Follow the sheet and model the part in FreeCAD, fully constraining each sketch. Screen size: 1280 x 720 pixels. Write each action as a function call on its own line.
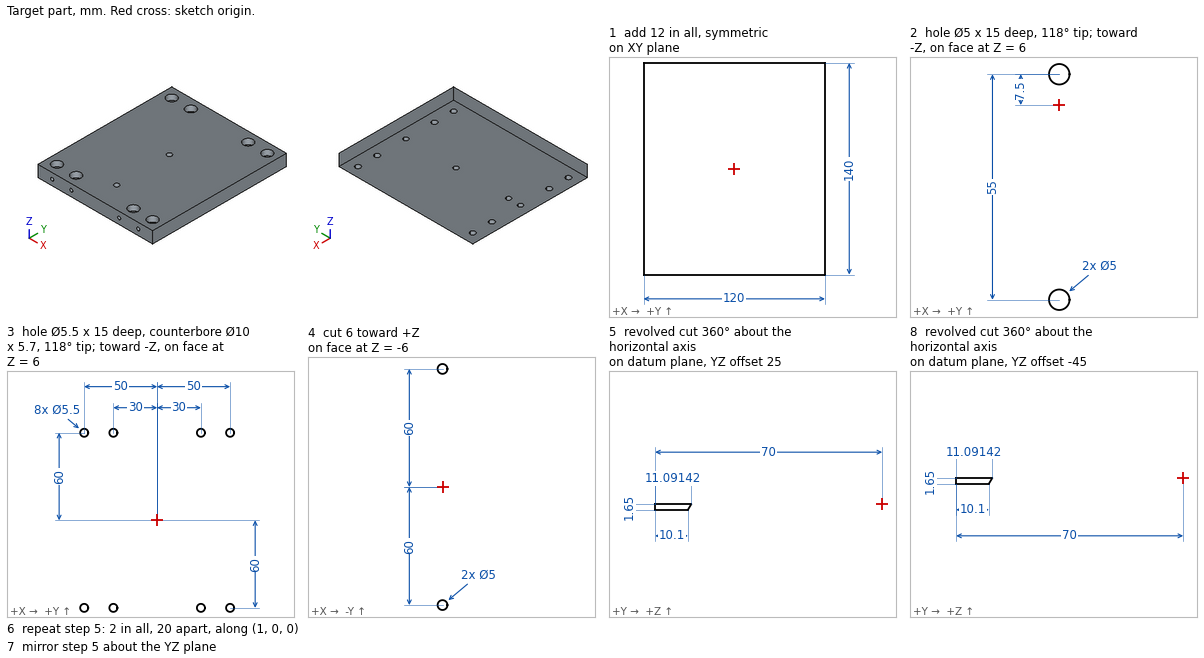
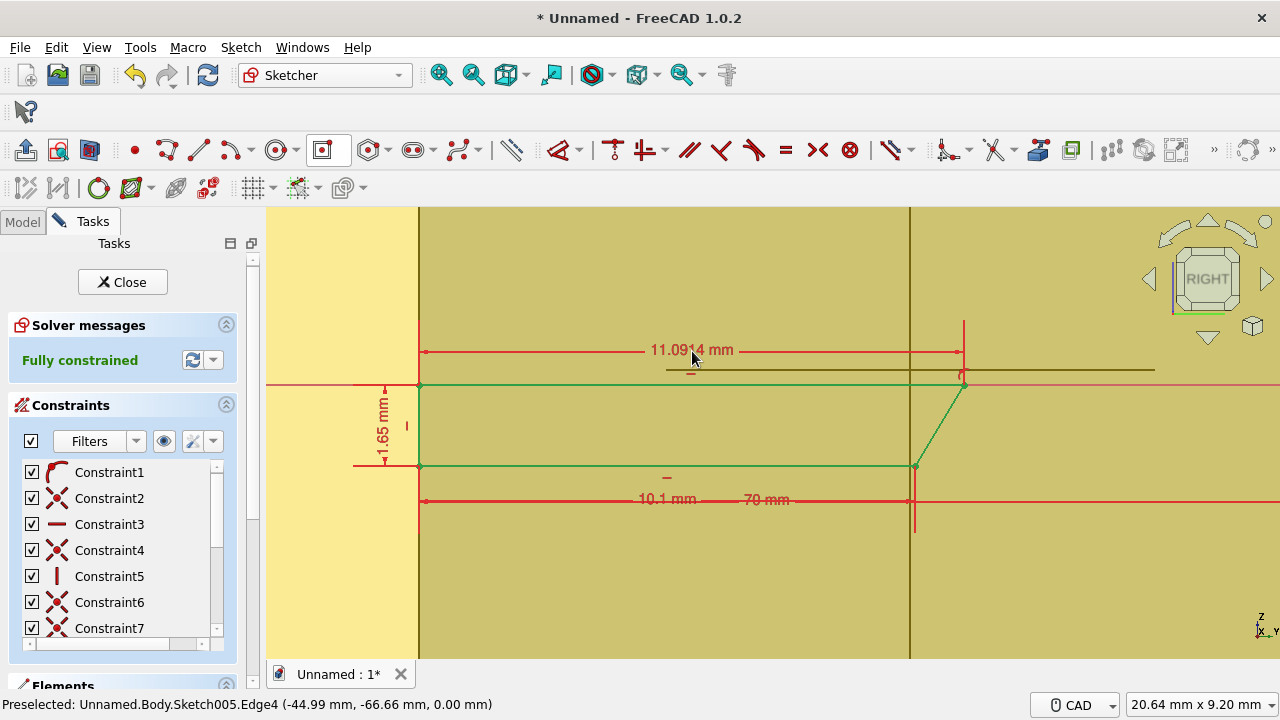
click(123, 282)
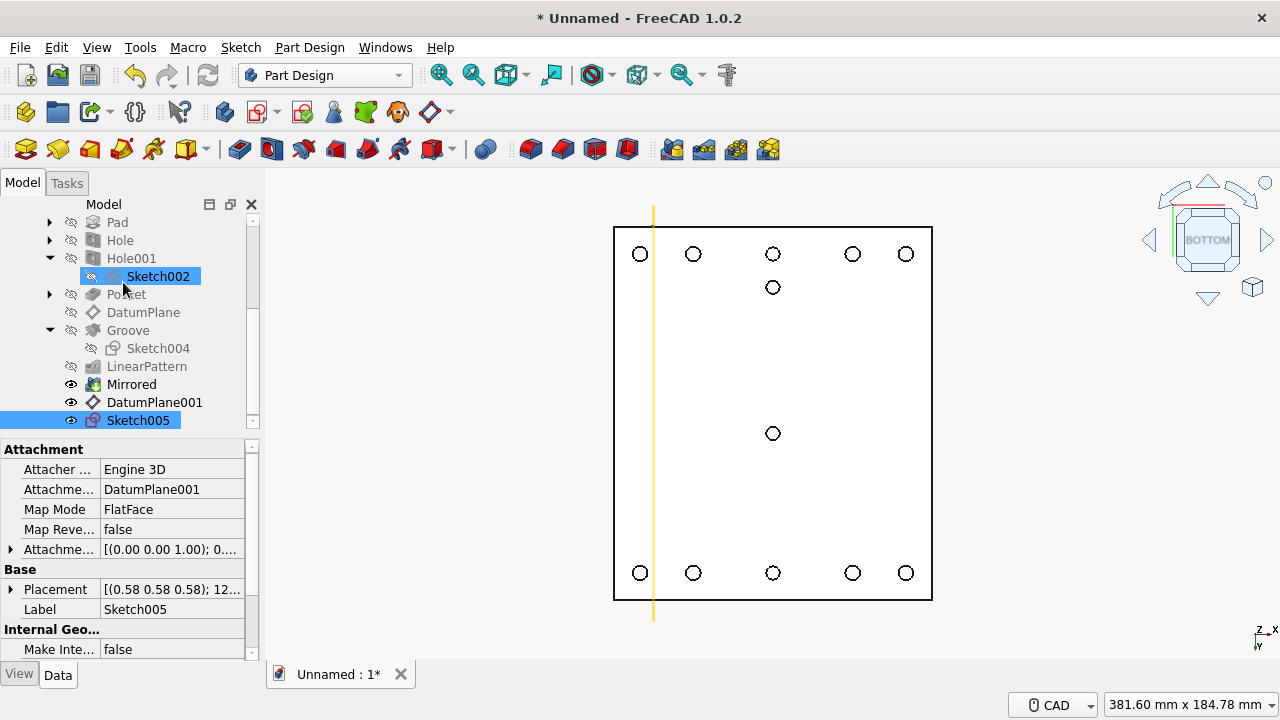
click(304, 150)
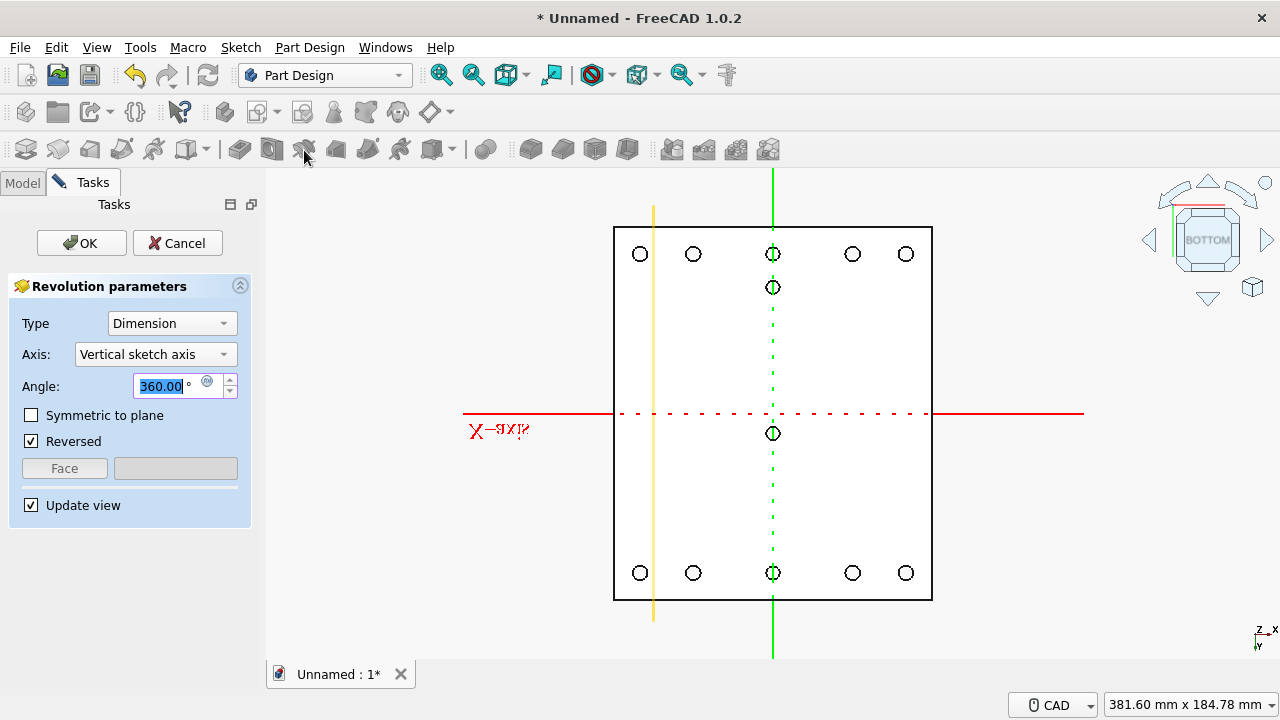
click(156, 354)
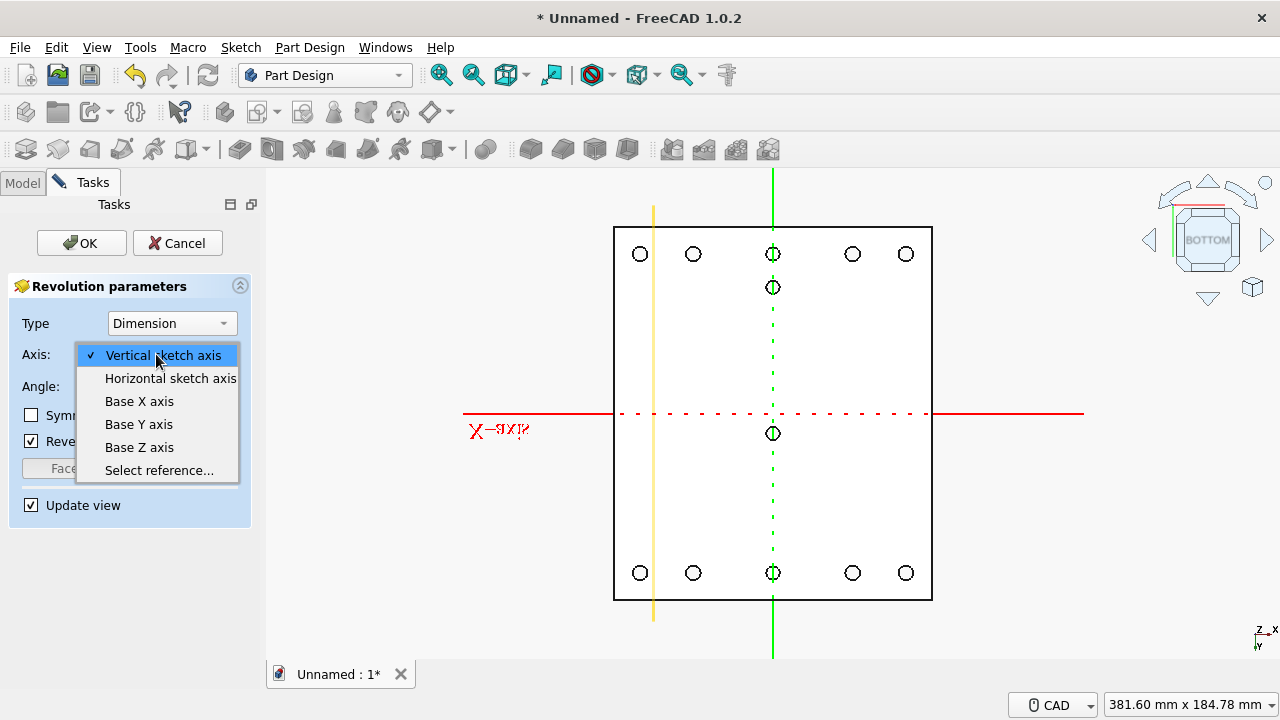
click(156, 378)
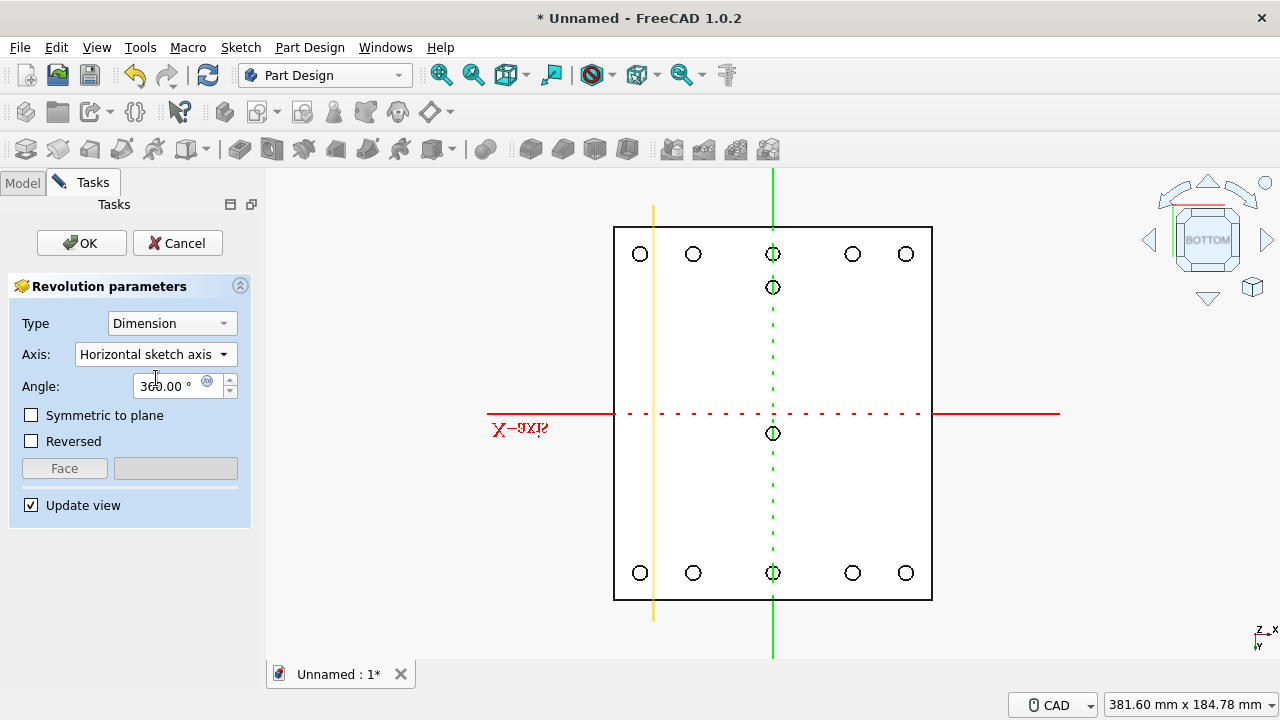
click(82, 243)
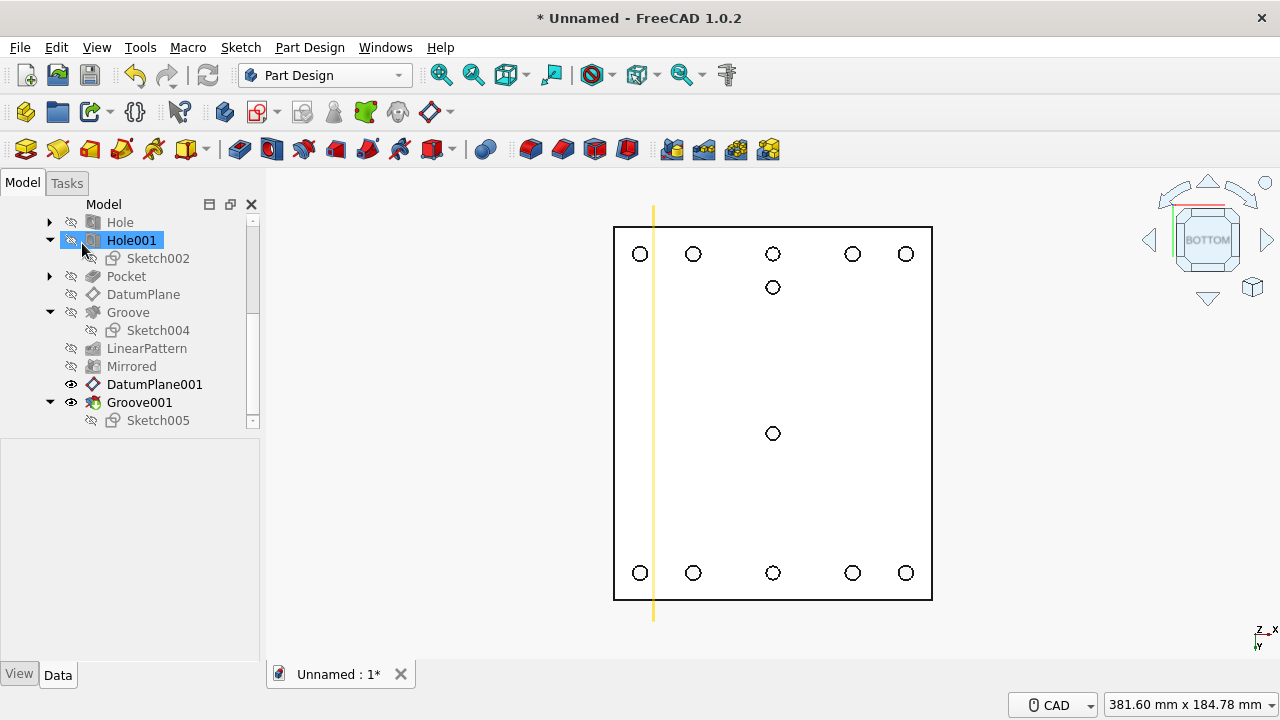
click(116, 384)
key(space)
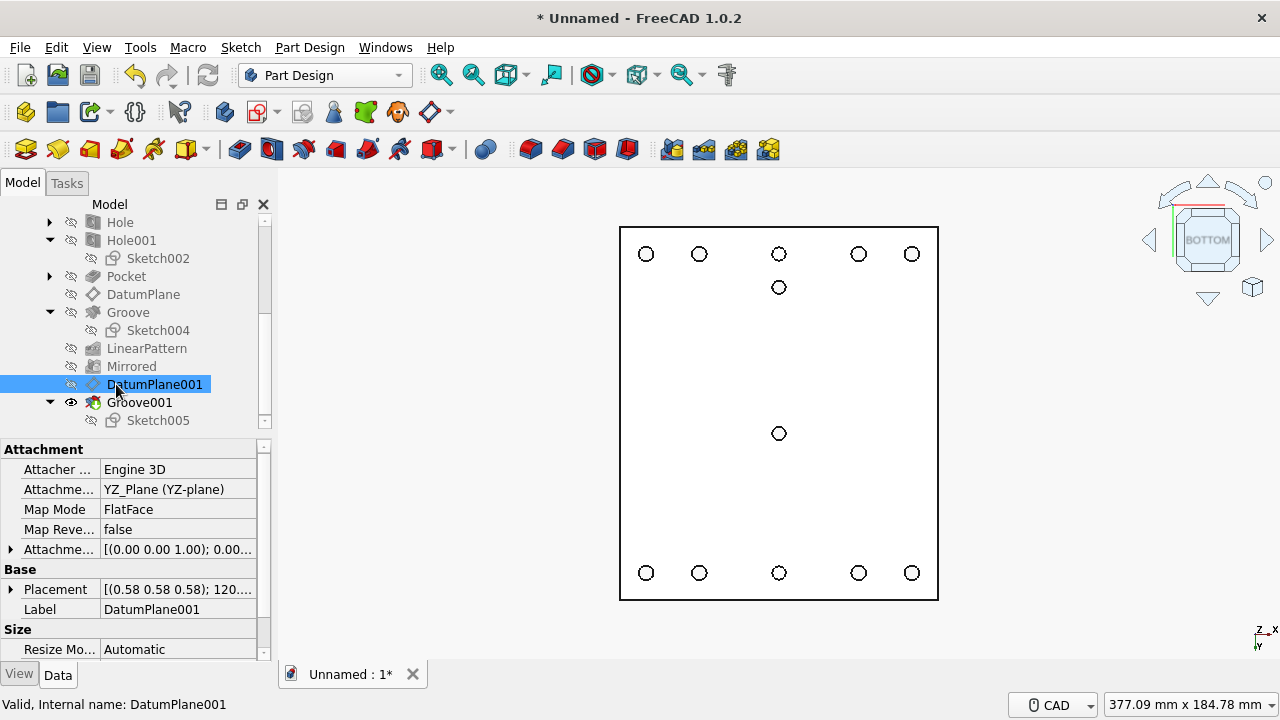
key(0)